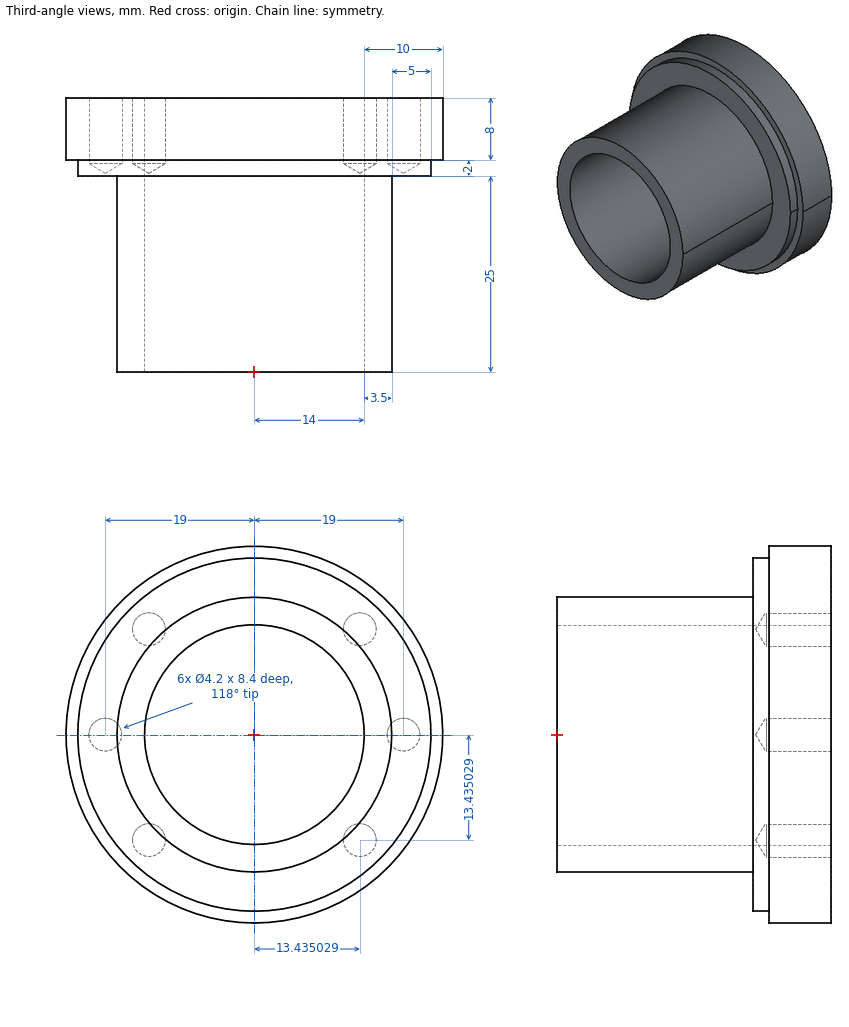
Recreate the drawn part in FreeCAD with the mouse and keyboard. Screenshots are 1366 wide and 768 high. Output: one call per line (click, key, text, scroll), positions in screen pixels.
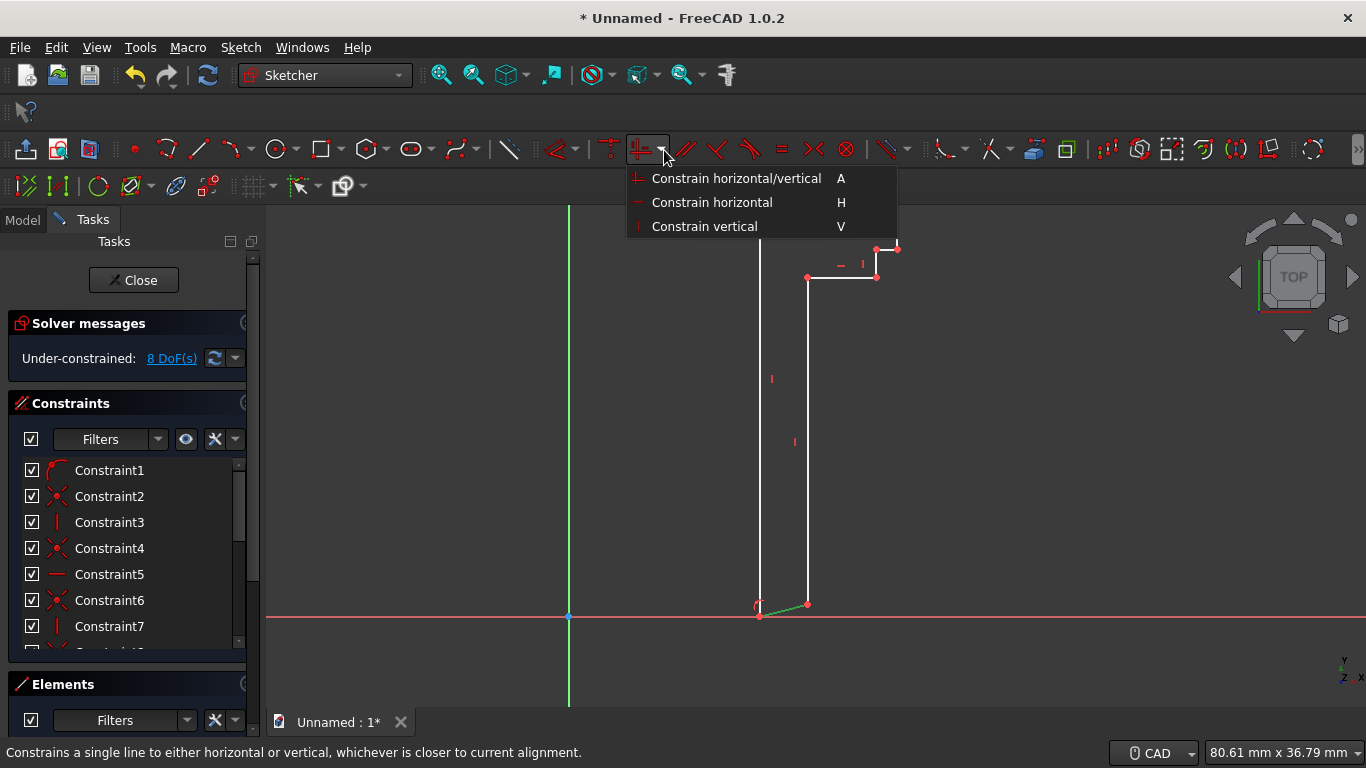
click(762, 202)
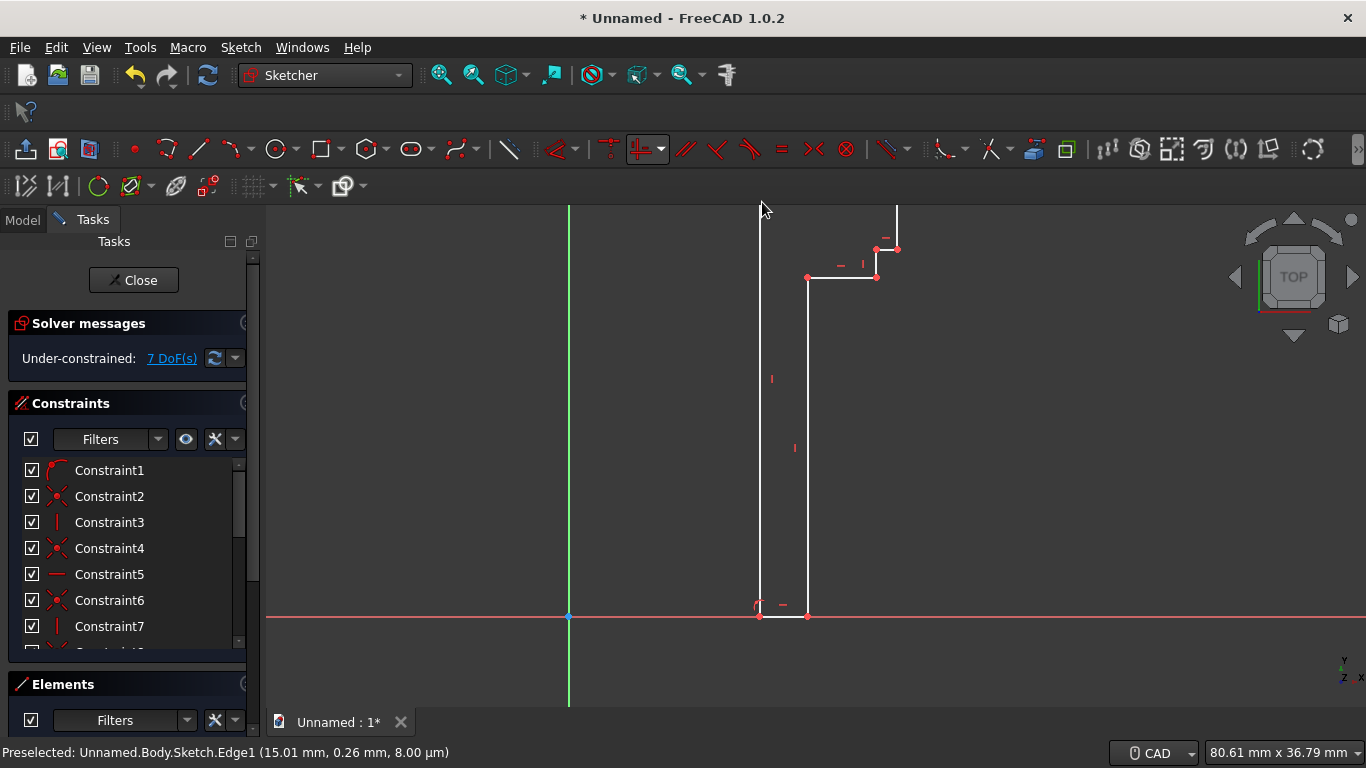
click(828, 278)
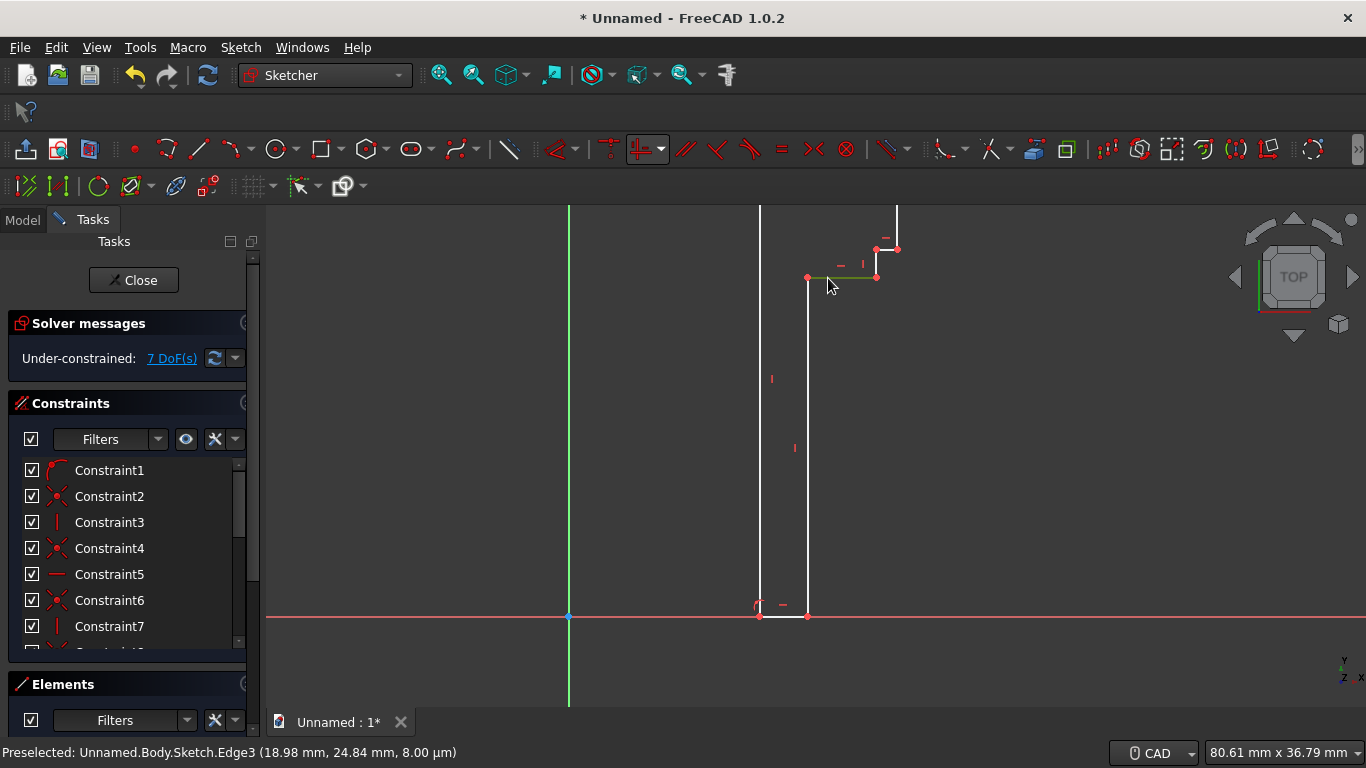
key(l)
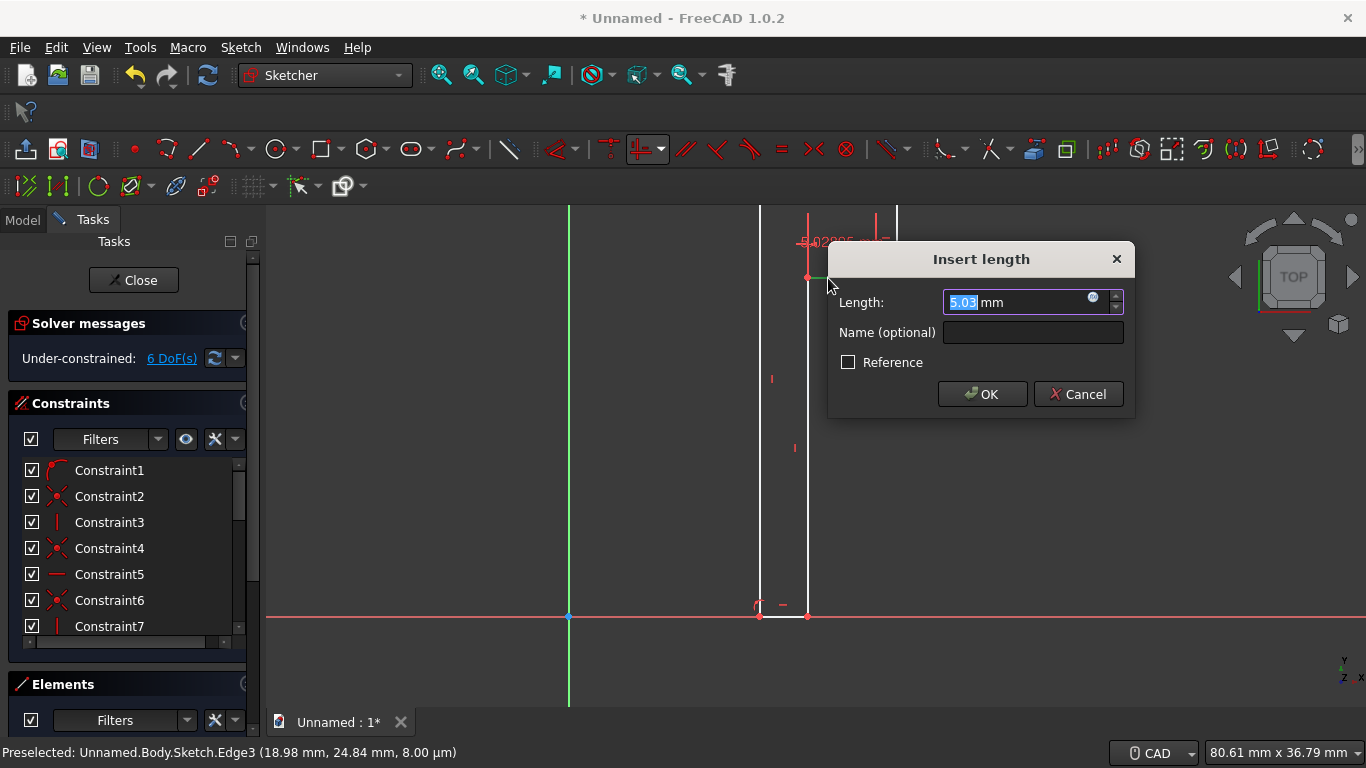
text(5)
key(Return)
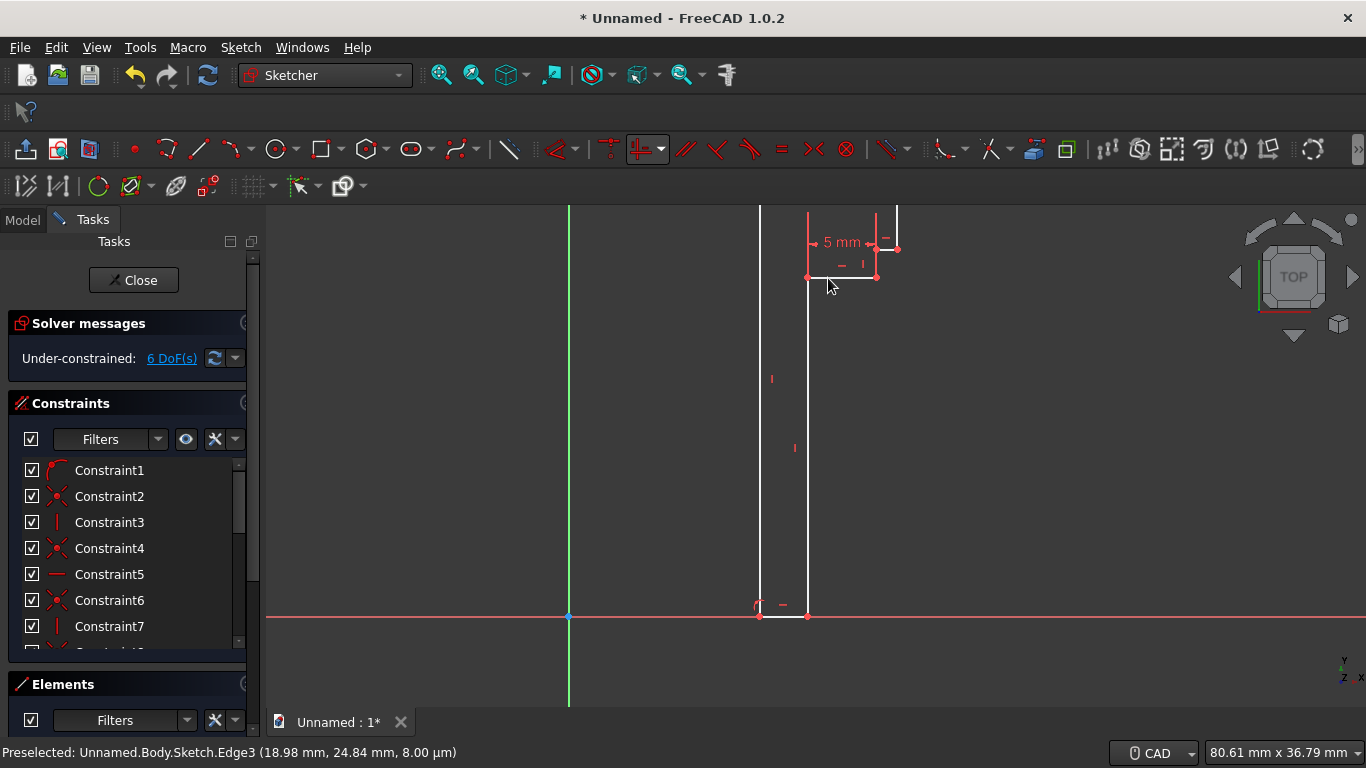
scroll(876, 267, up, 2)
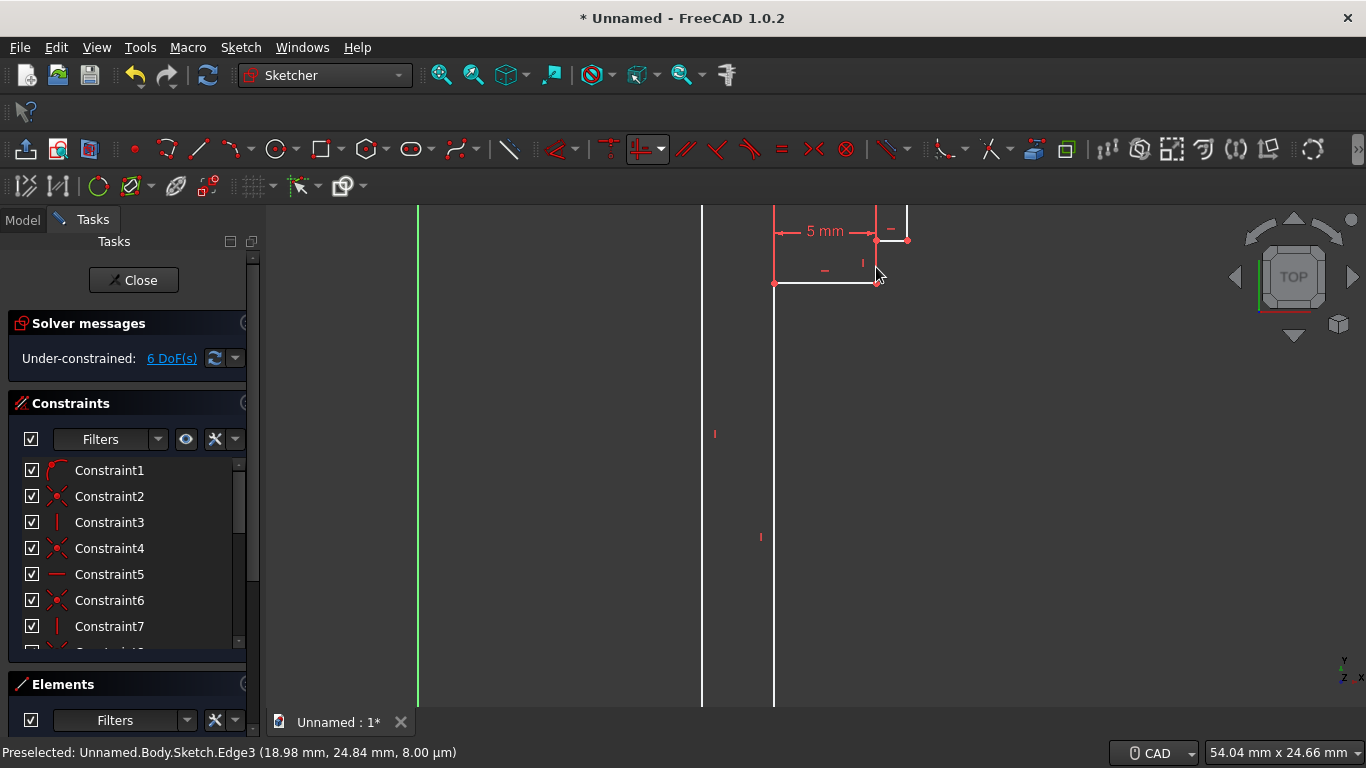
click(876, 266)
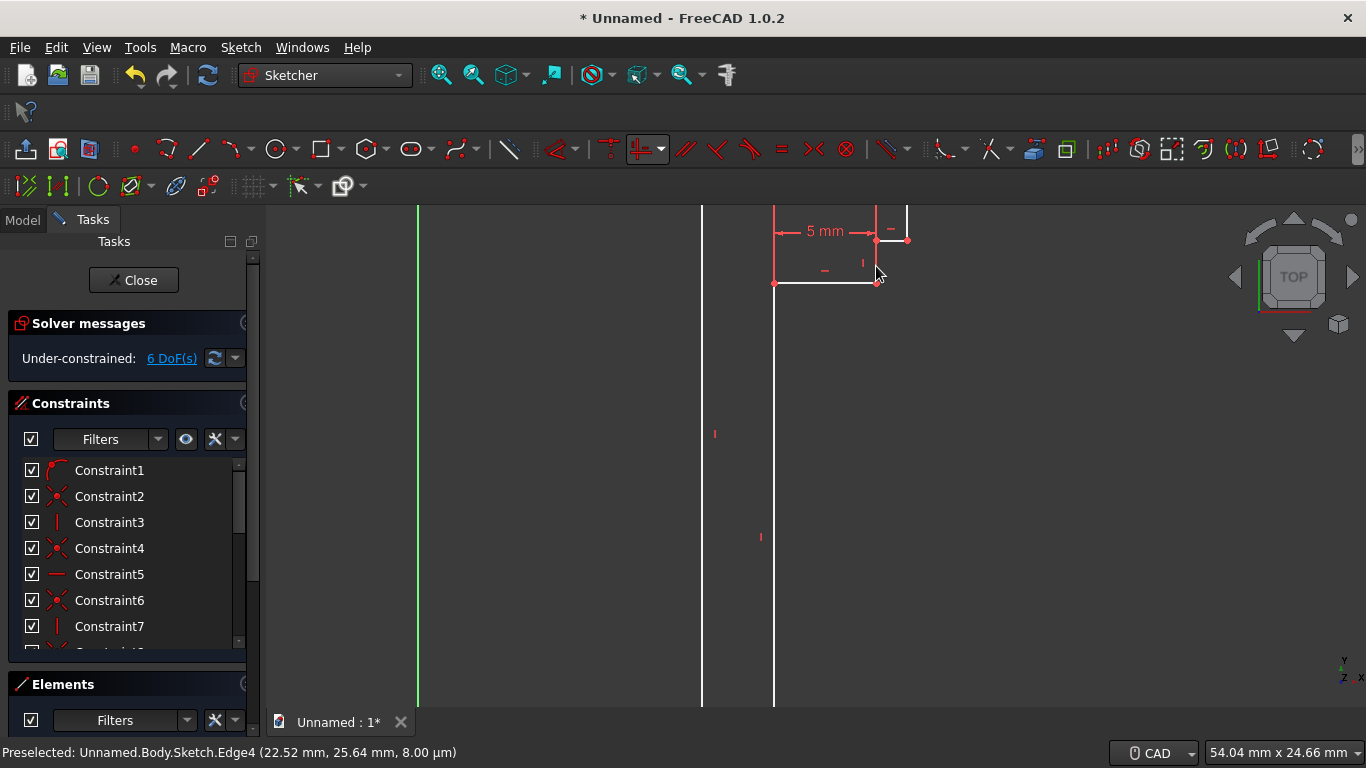
click(578, 150)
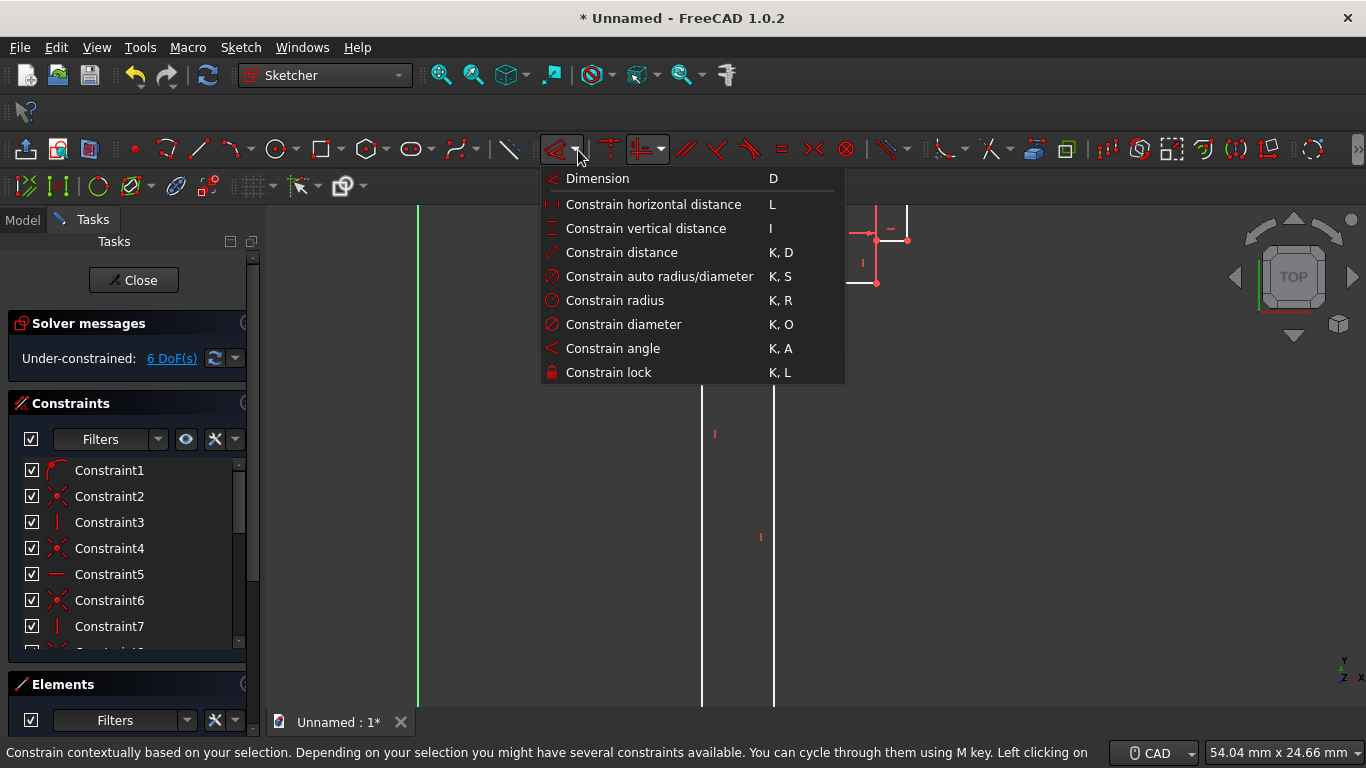
click(693, 228)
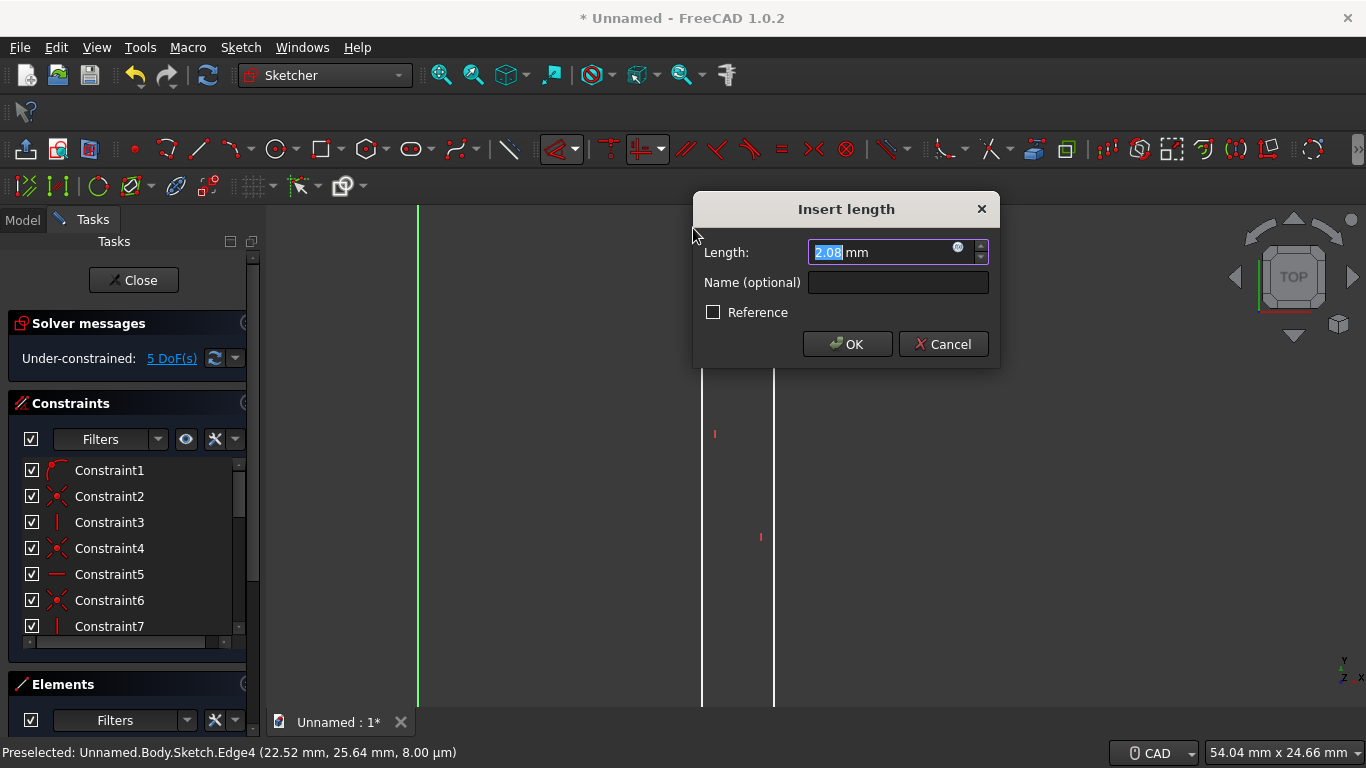
text(2)
key(Return)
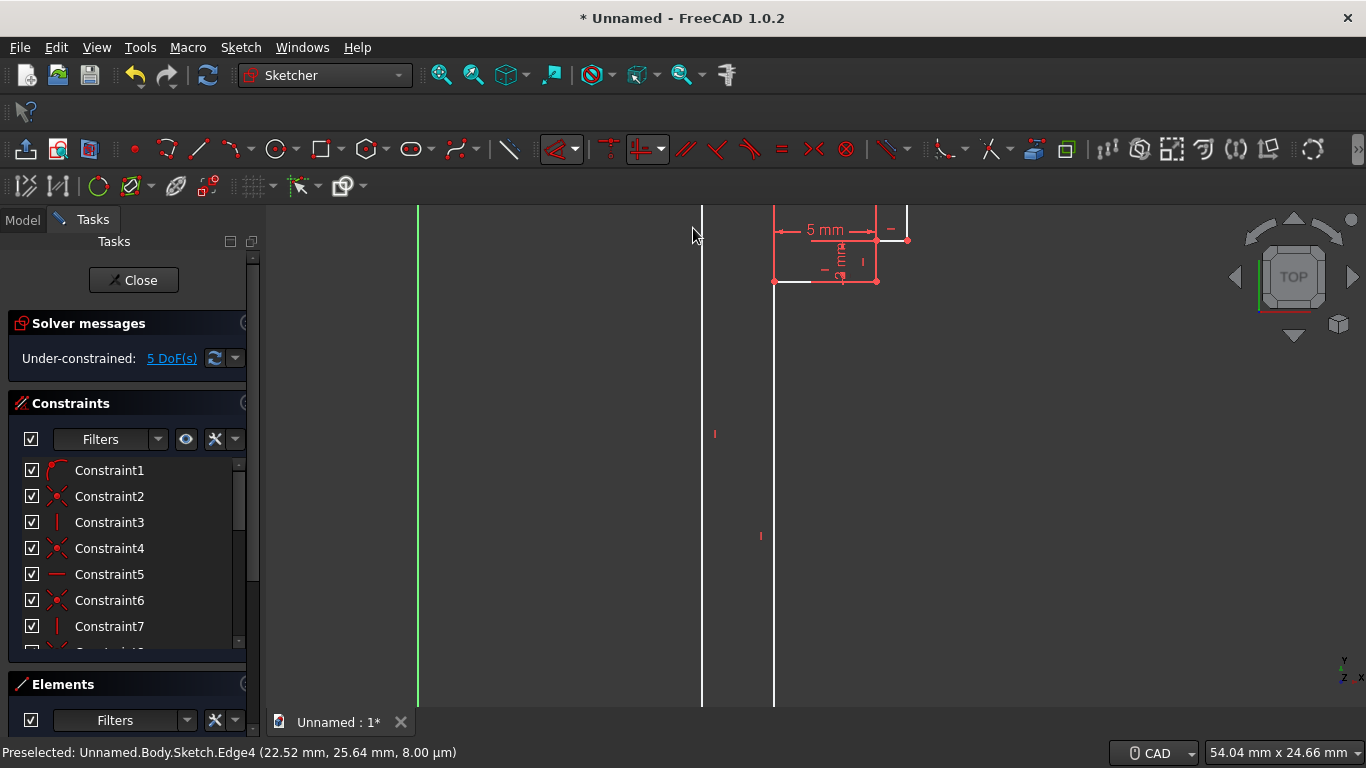
scroll(817, 475, down, 4)